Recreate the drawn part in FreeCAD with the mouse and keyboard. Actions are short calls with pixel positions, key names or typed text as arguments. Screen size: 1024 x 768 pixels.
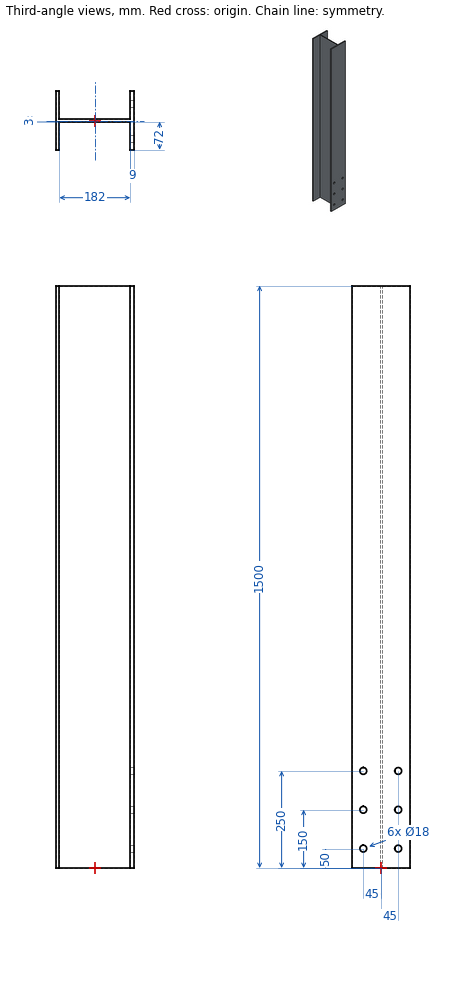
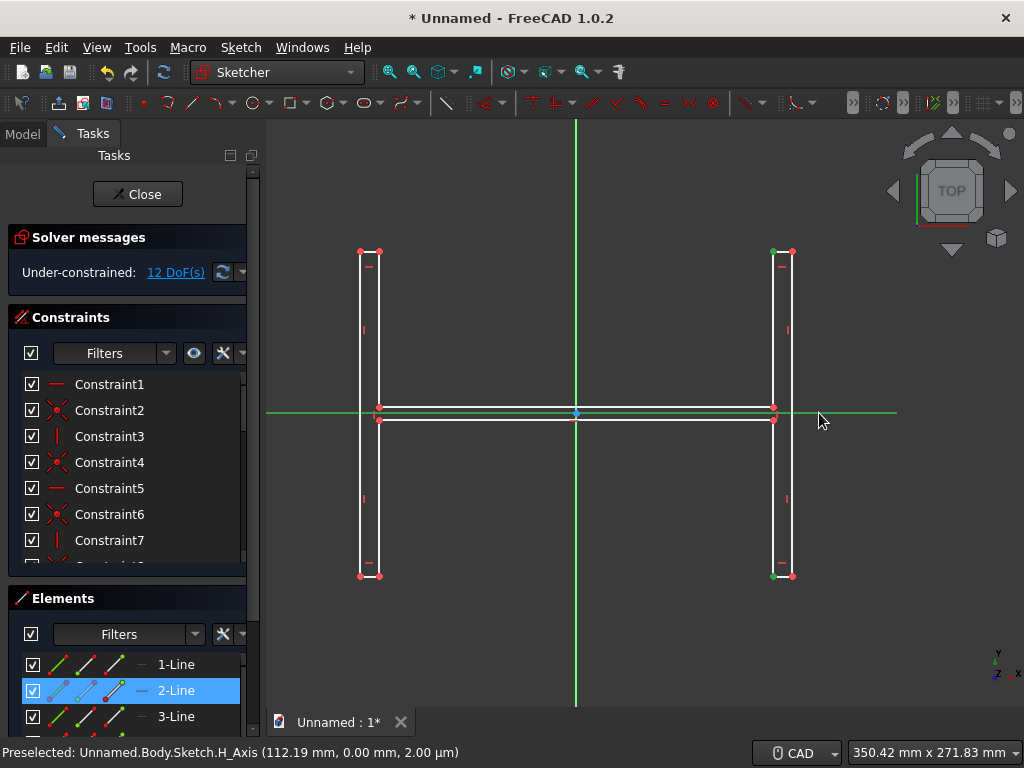
key(s)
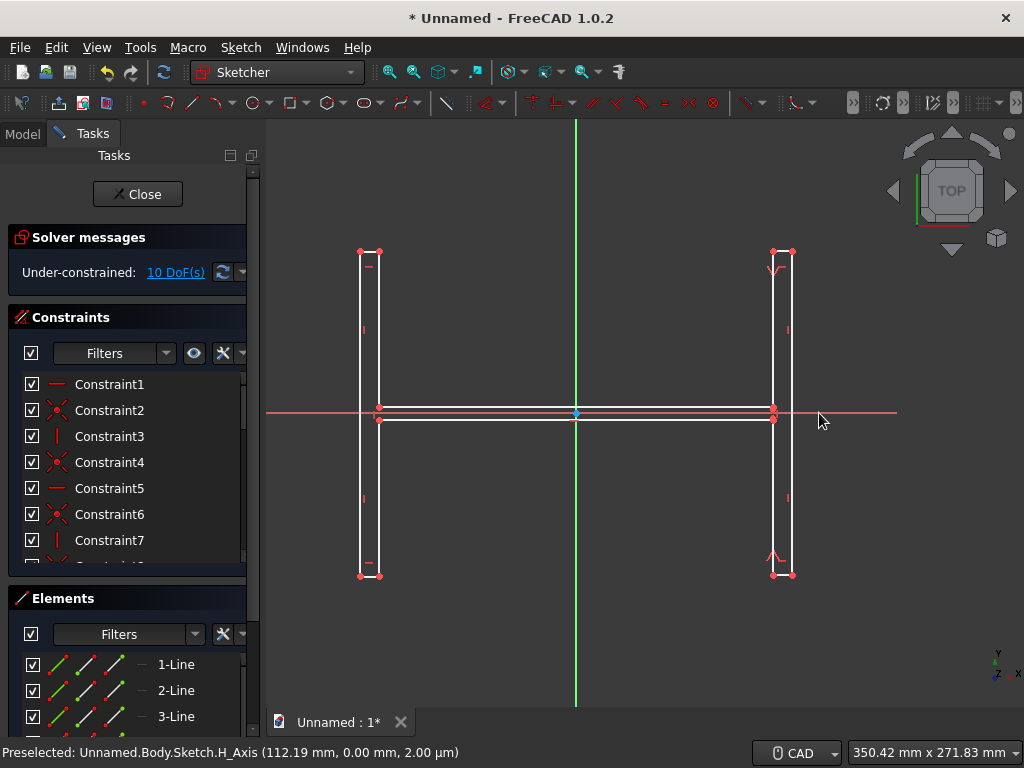
click(379, 420)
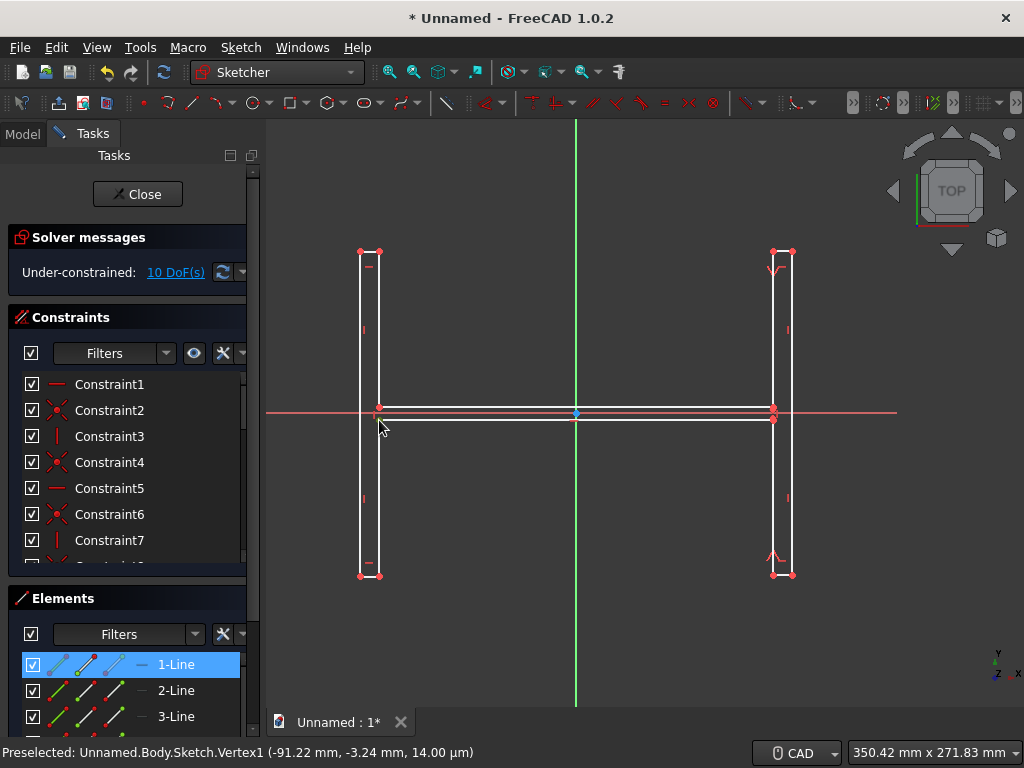
click(379, 407)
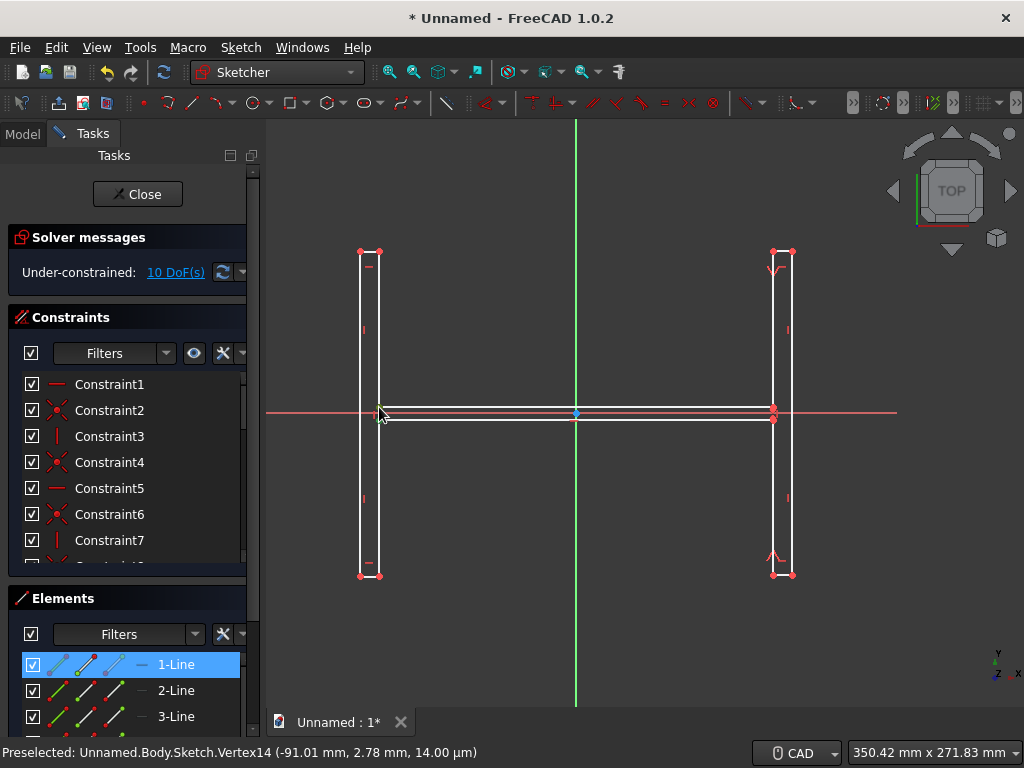
click(819, 413)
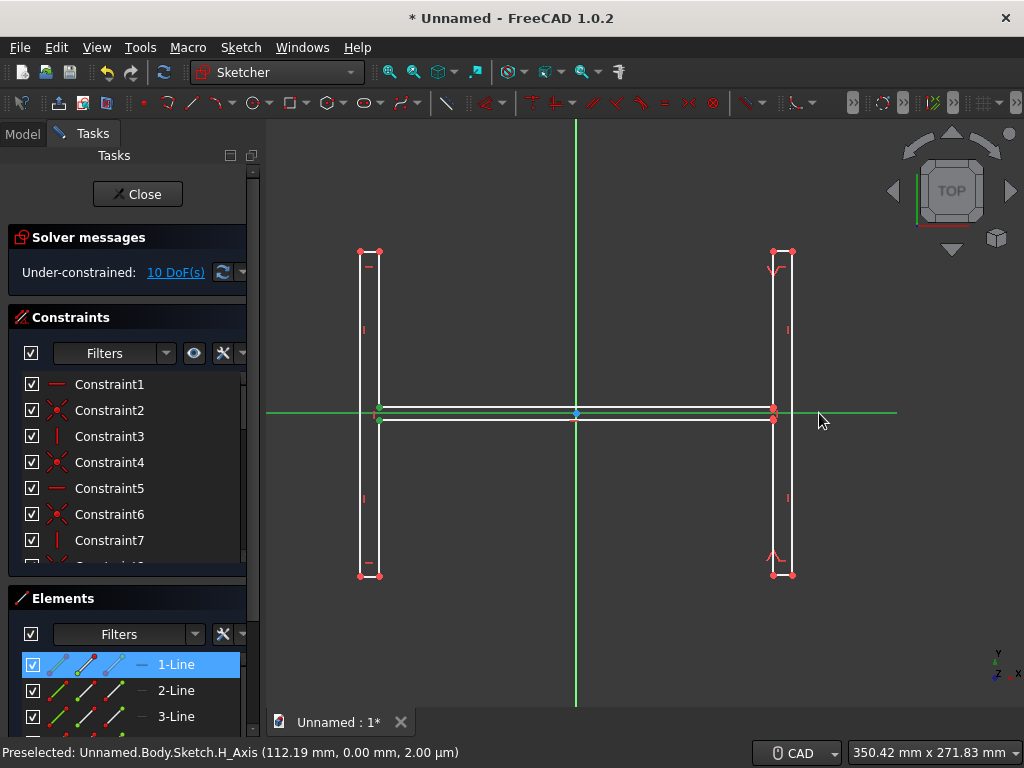
click(690, 104)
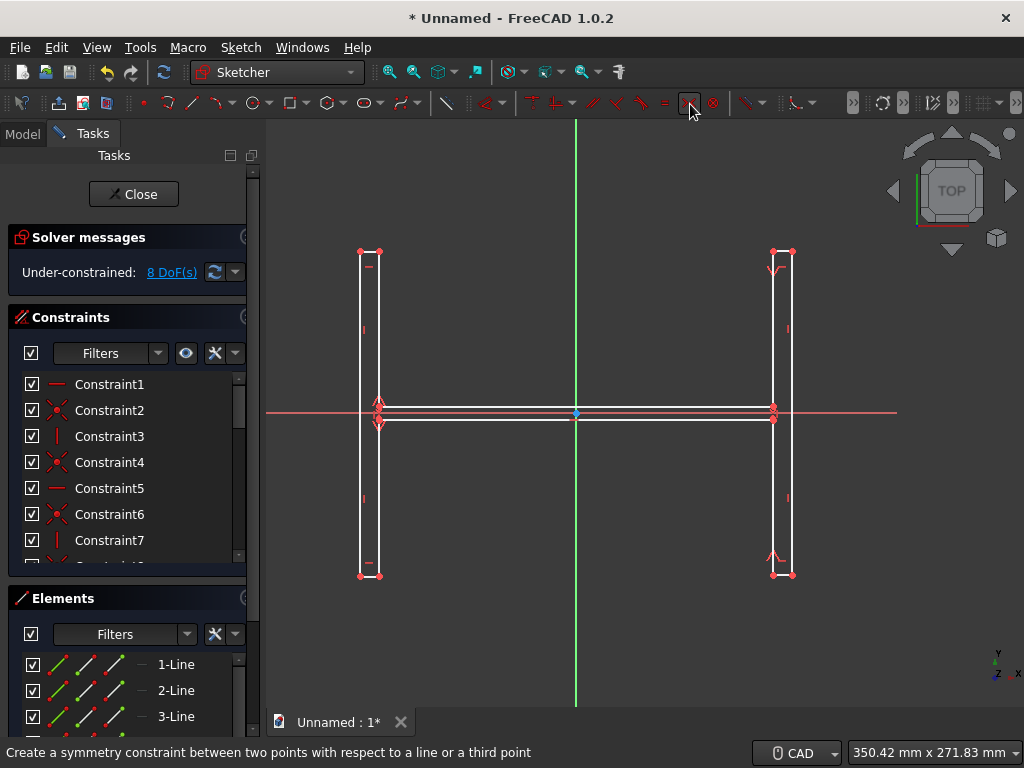
click(773, 251)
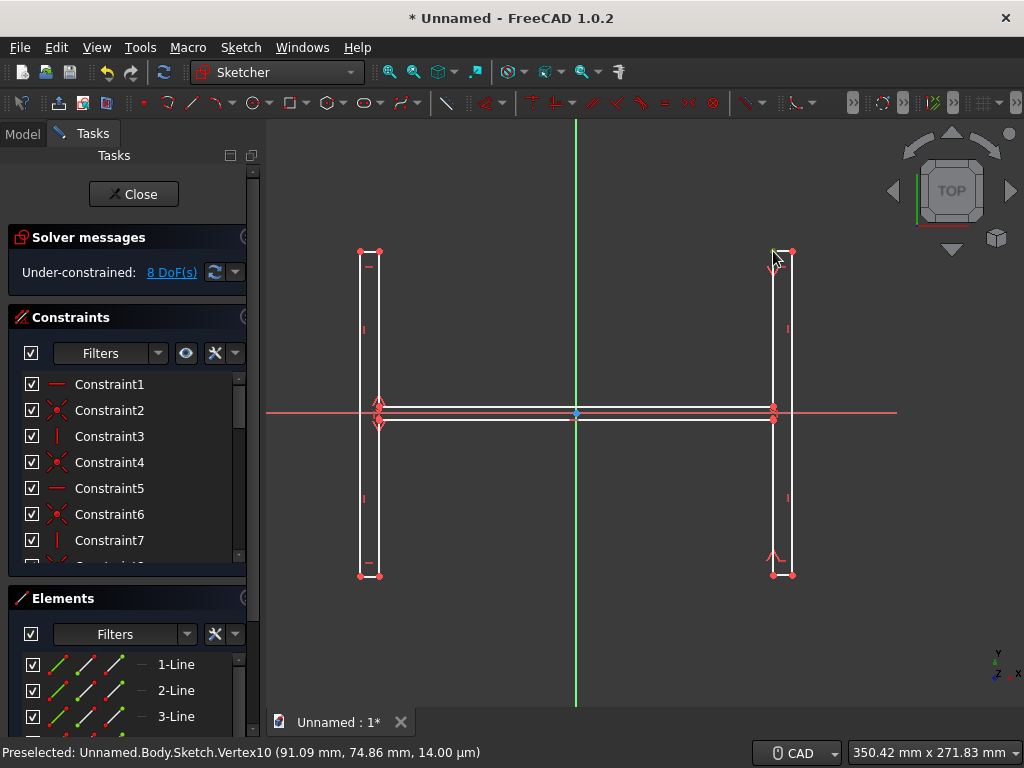
click(379, 252)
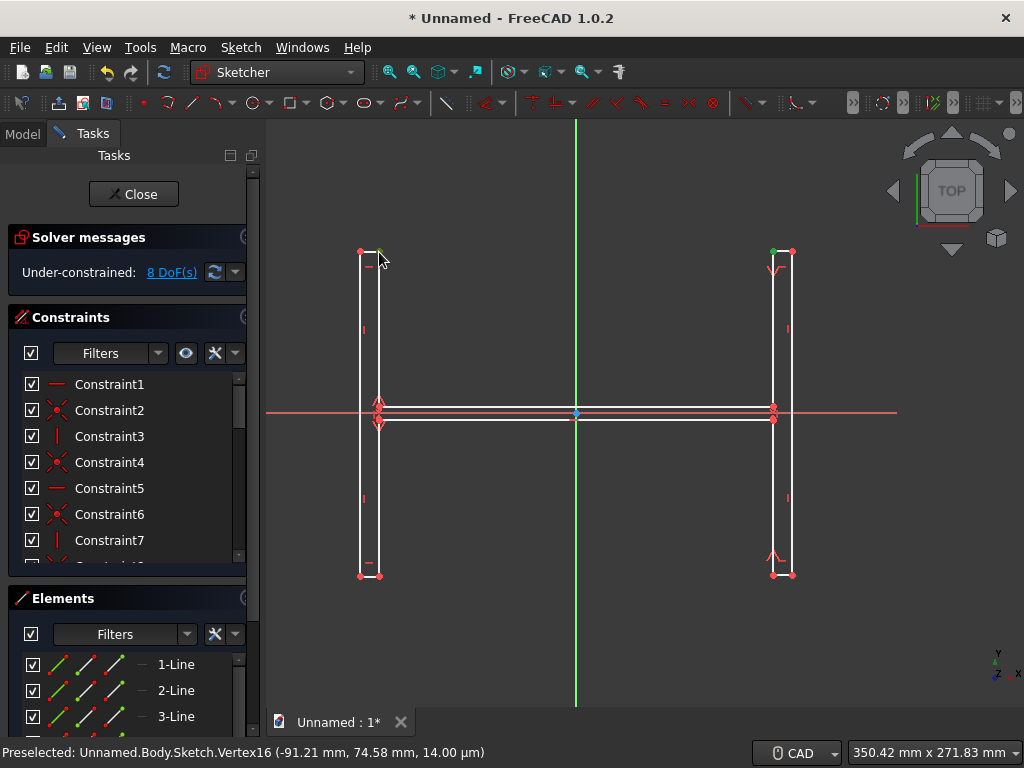
click(576, 641)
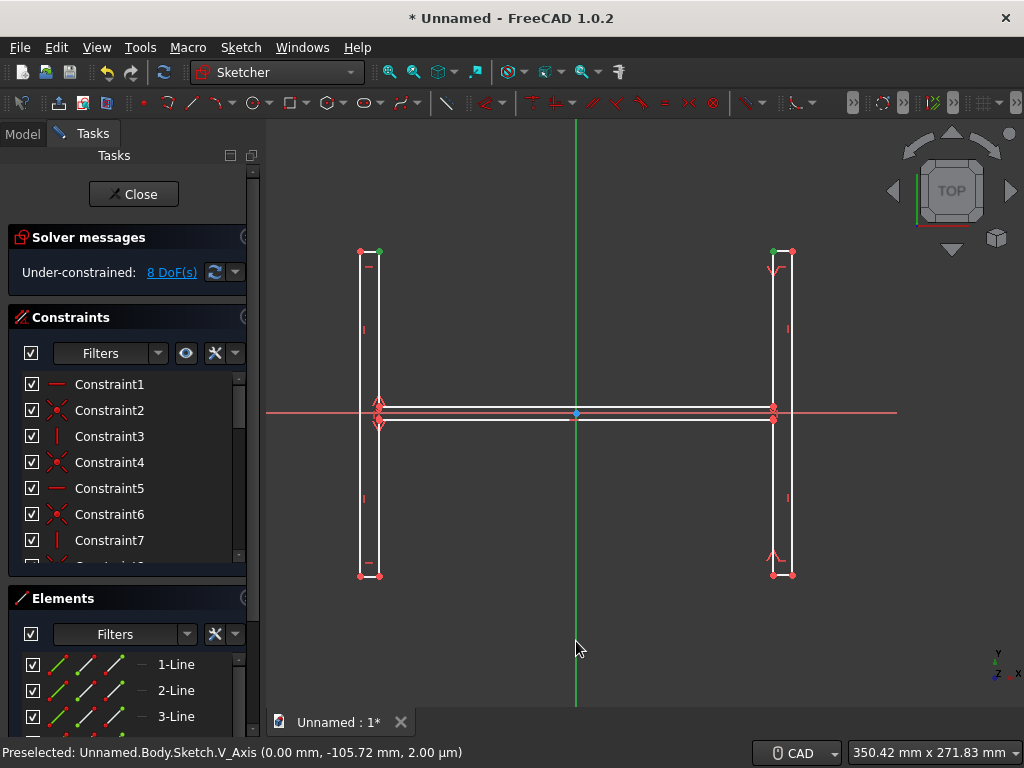
click(690, 104)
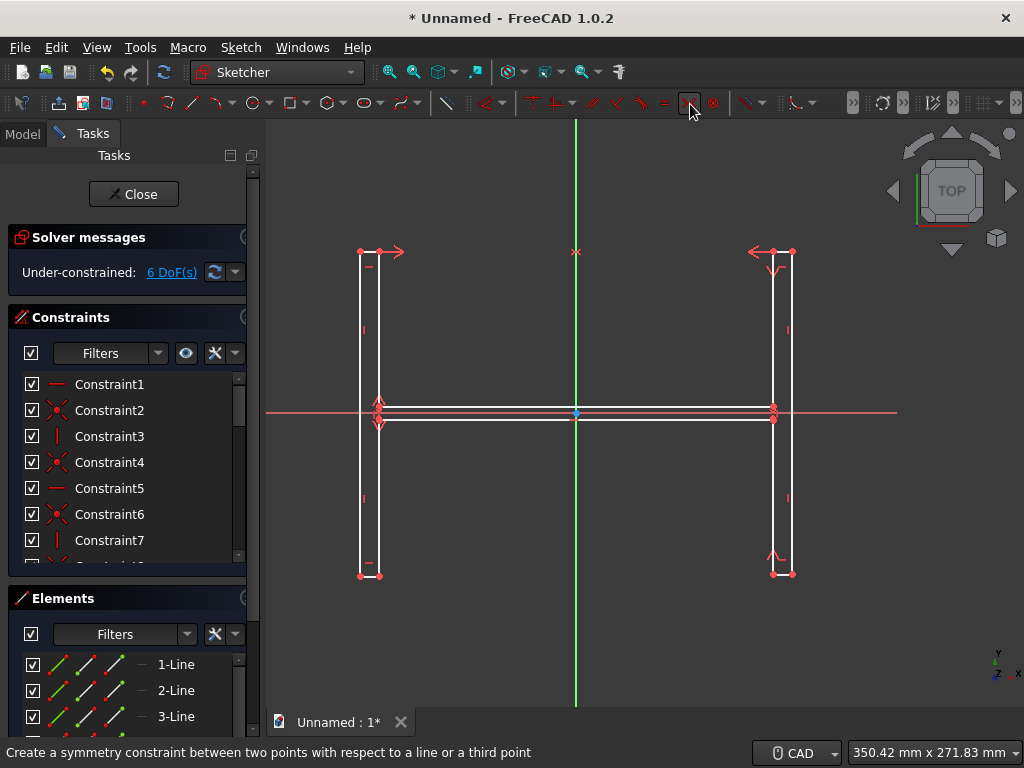
click(792, 575)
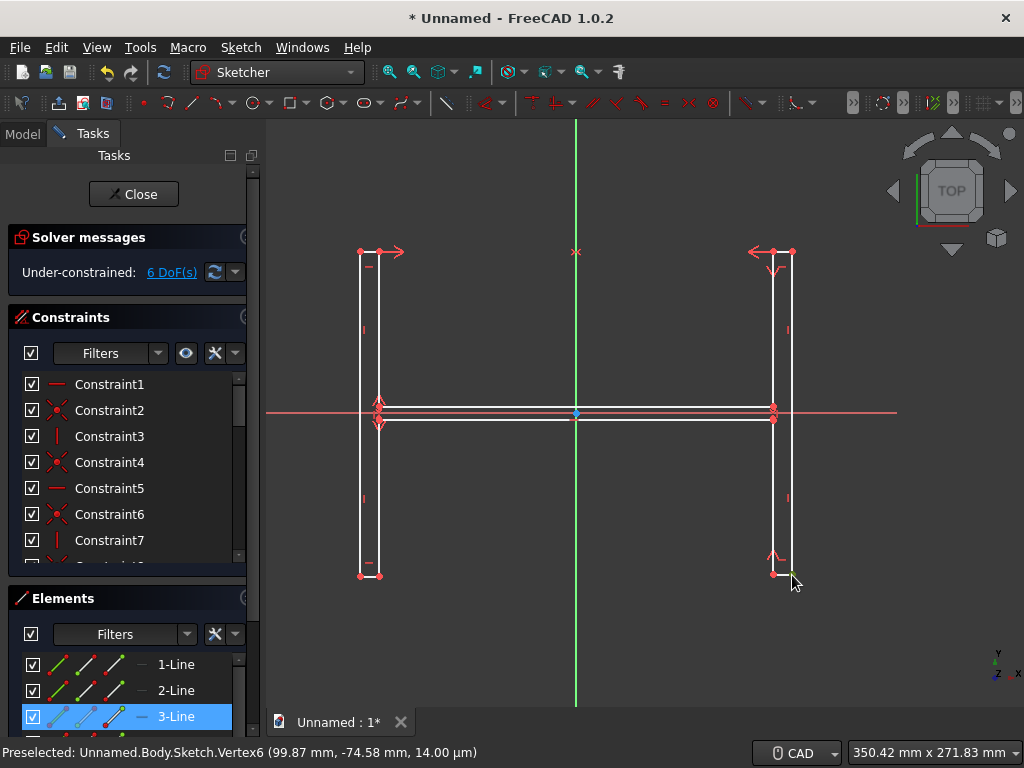
click(360, 577)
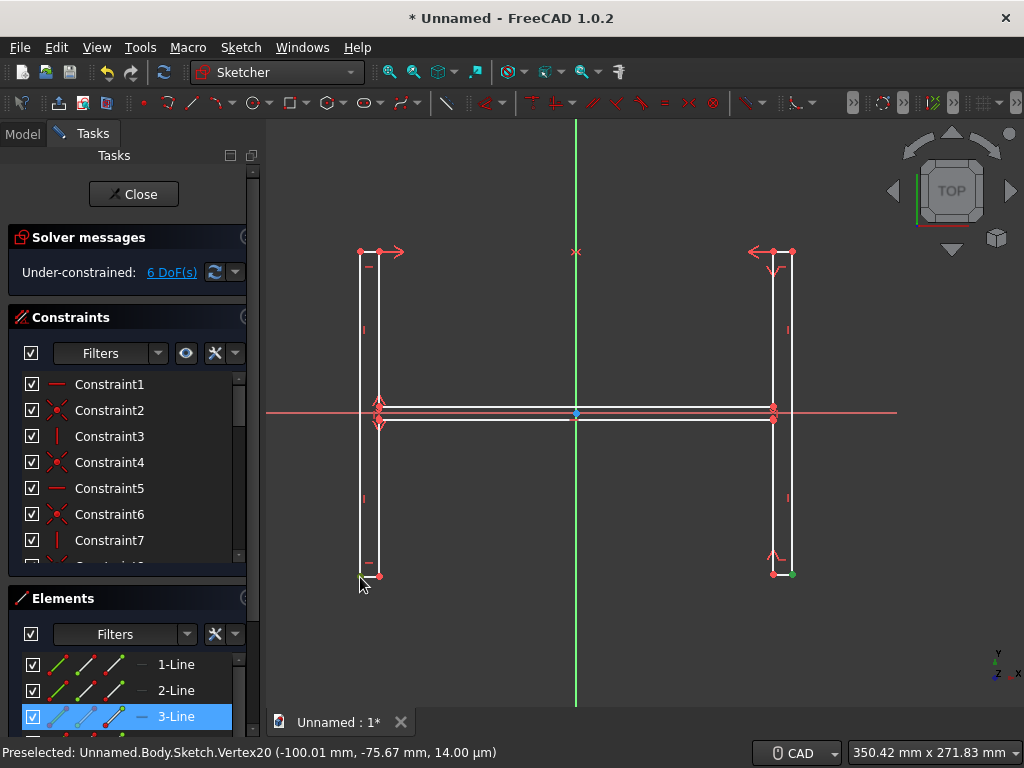
click(576, 641)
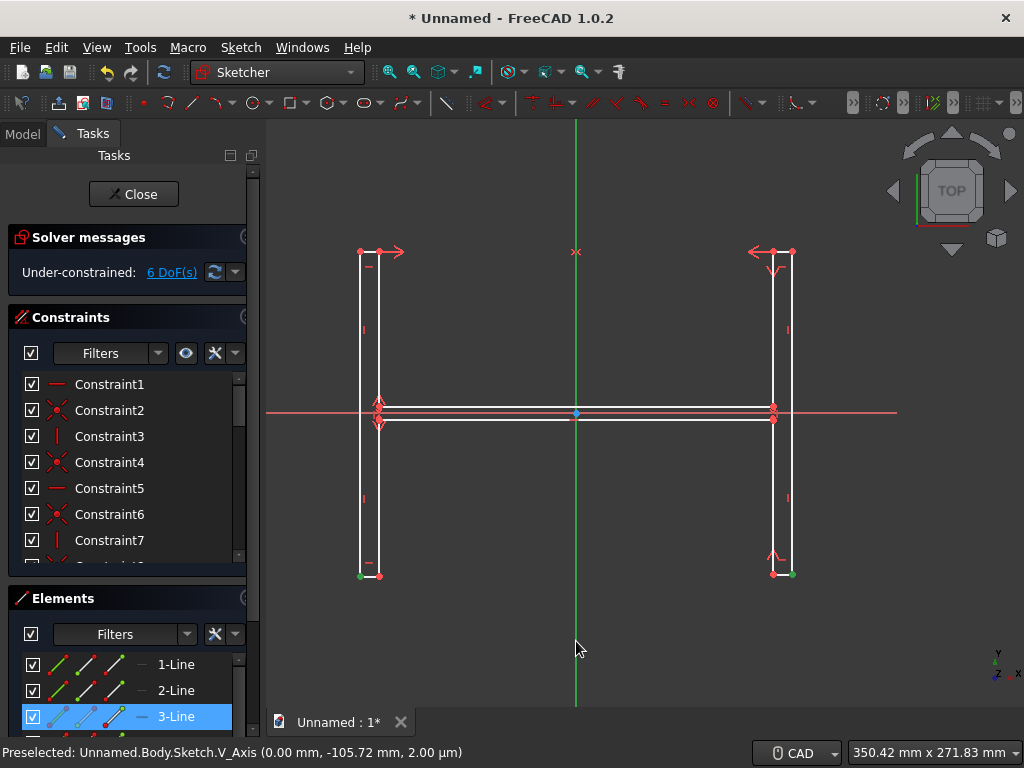
click(690, 104)